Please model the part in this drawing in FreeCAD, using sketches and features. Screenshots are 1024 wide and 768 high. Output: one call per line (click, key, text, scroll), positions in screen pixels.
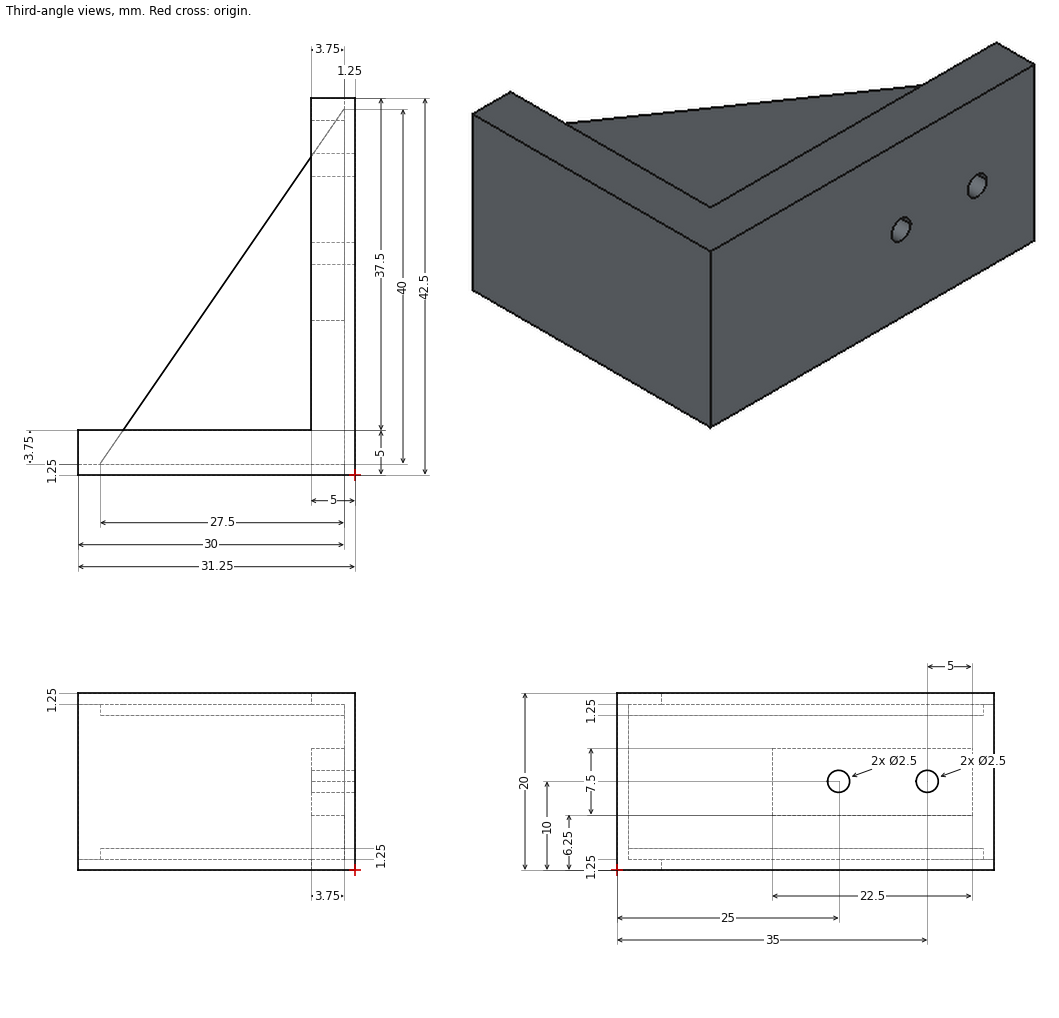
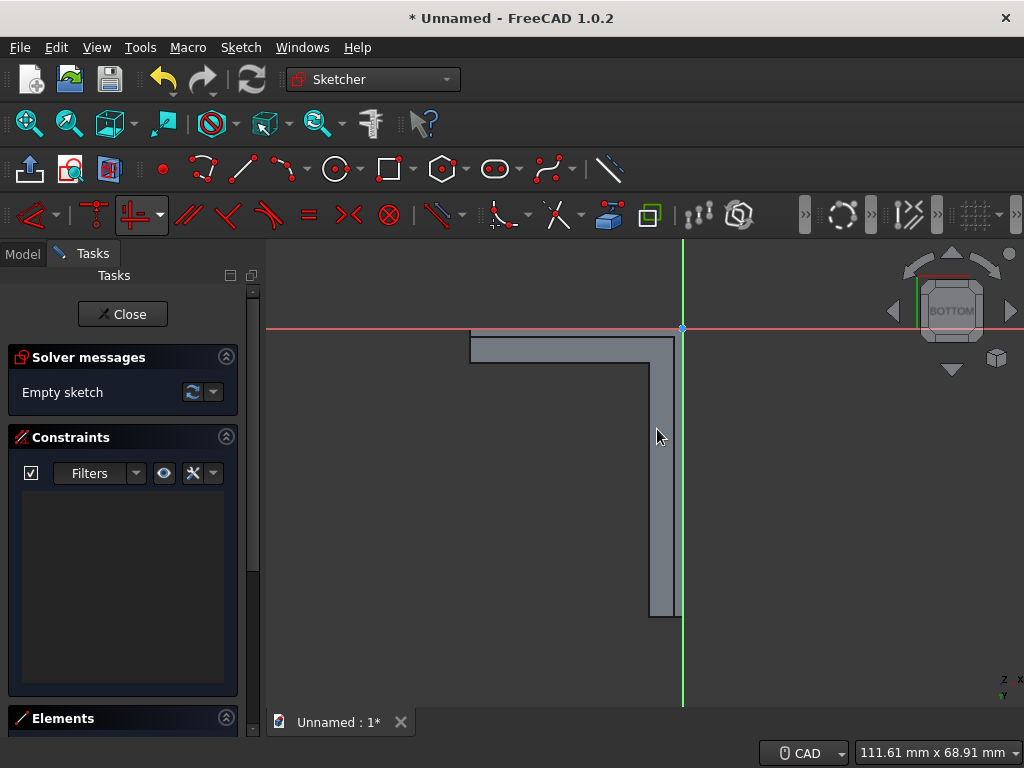
click(204, 170)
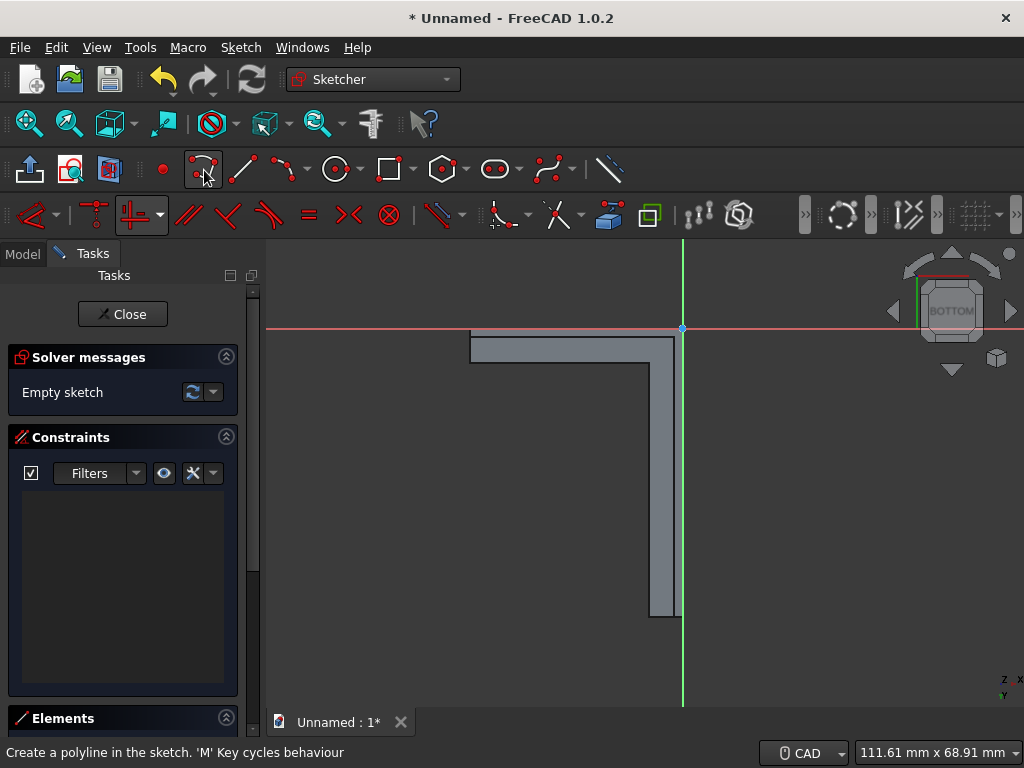
click(683, 329)
click(470, 338)
click(470, 363)
click(649, 363)
click(649, 617)
click(674, 617)
click(683, 329)
key(Escape)
key(Escape)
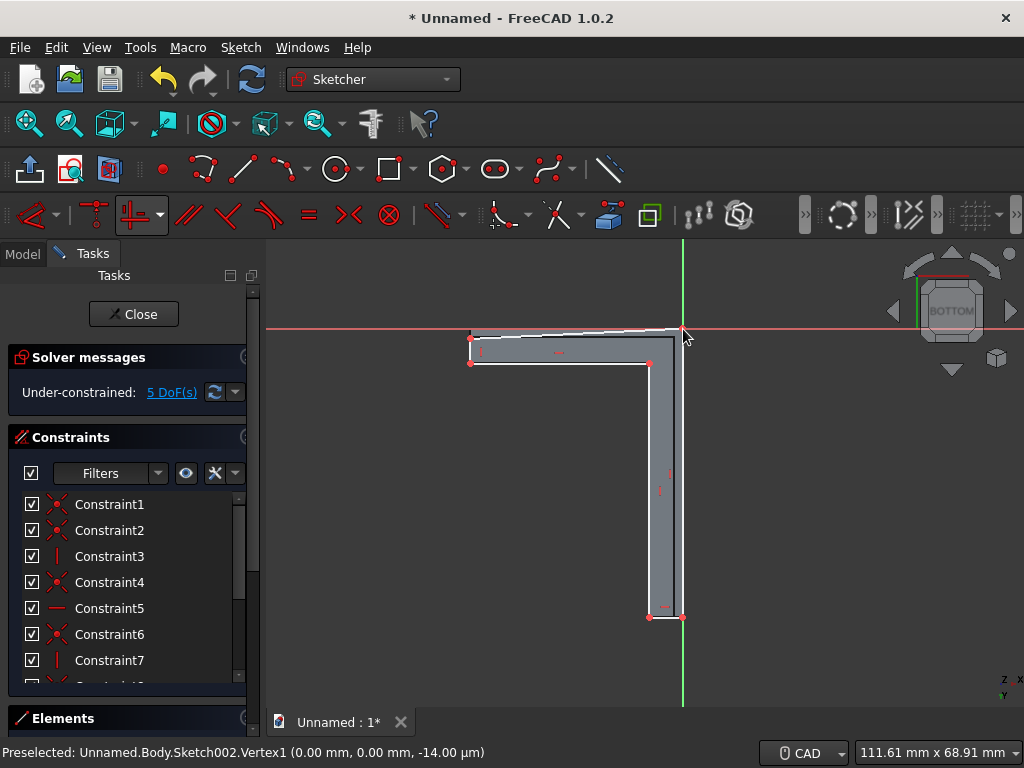
click(619, 332)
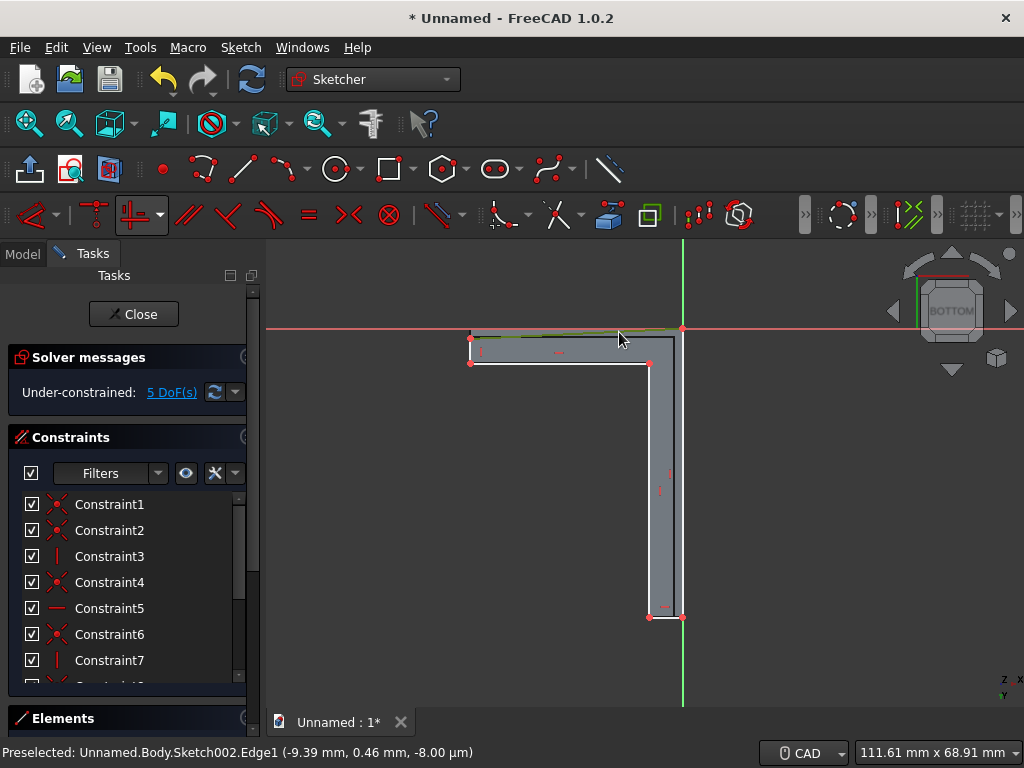
click(162, 216)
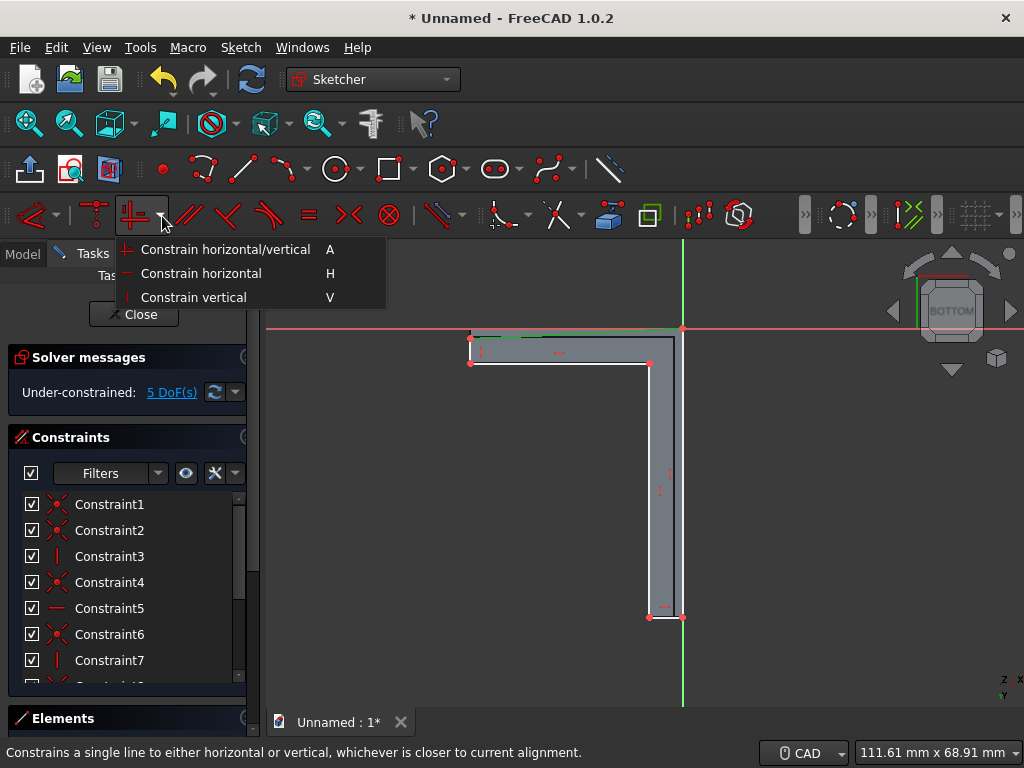
click(251, 273)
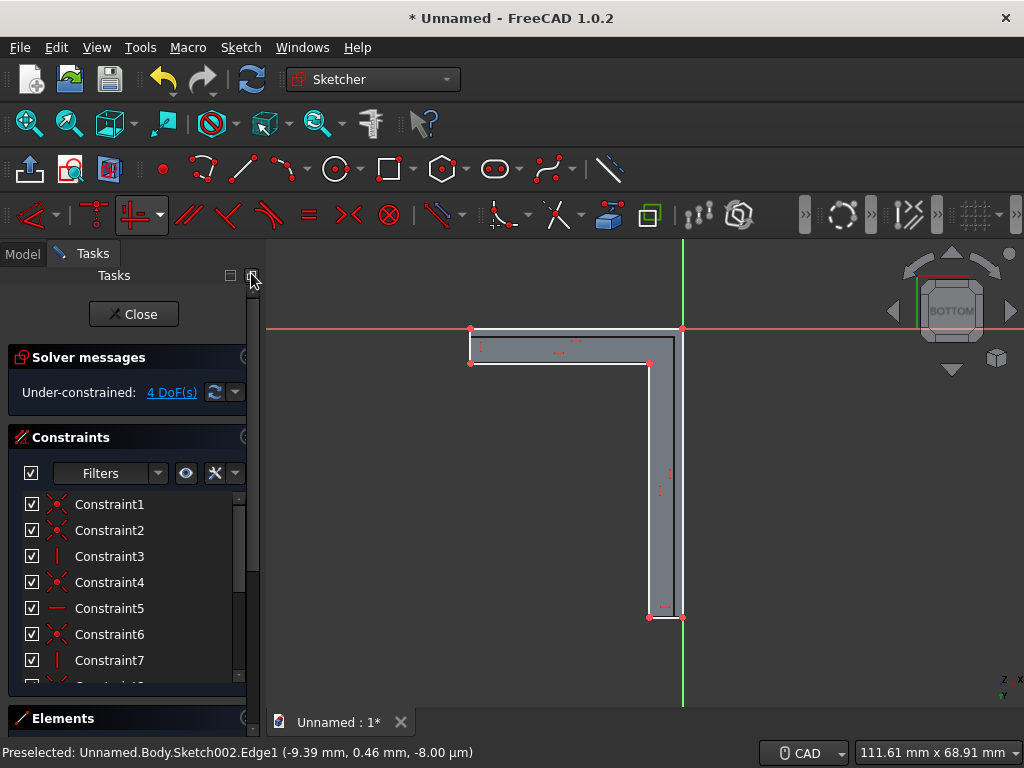
click(32, 216)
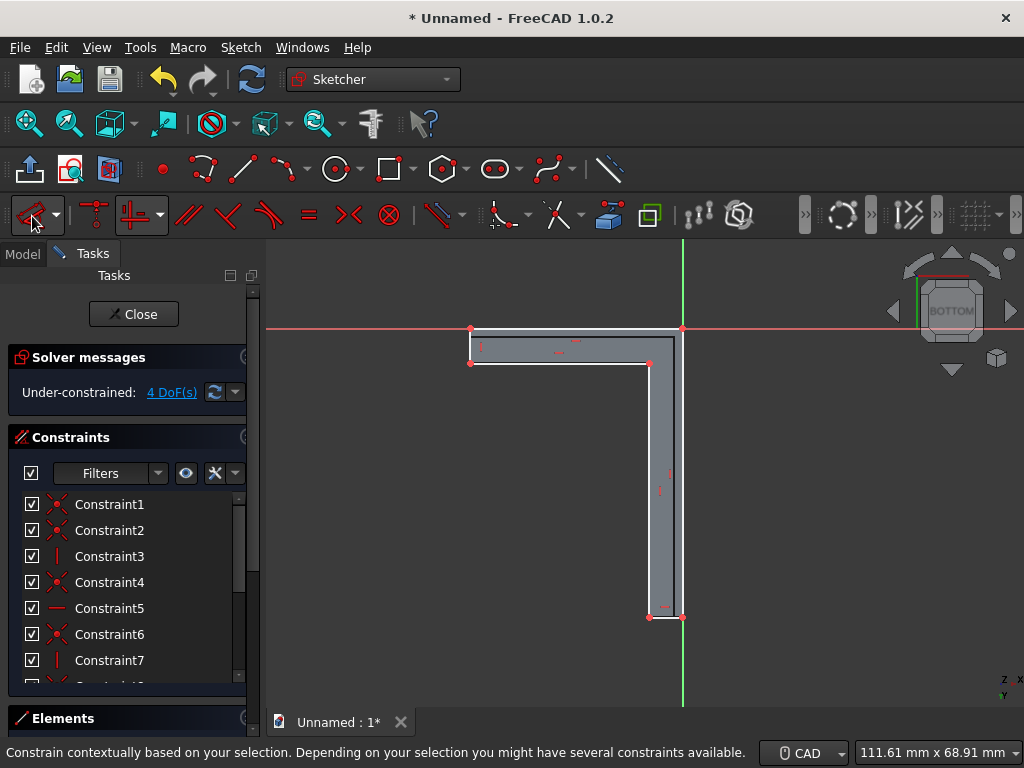
scroll(470, 339, up, 2)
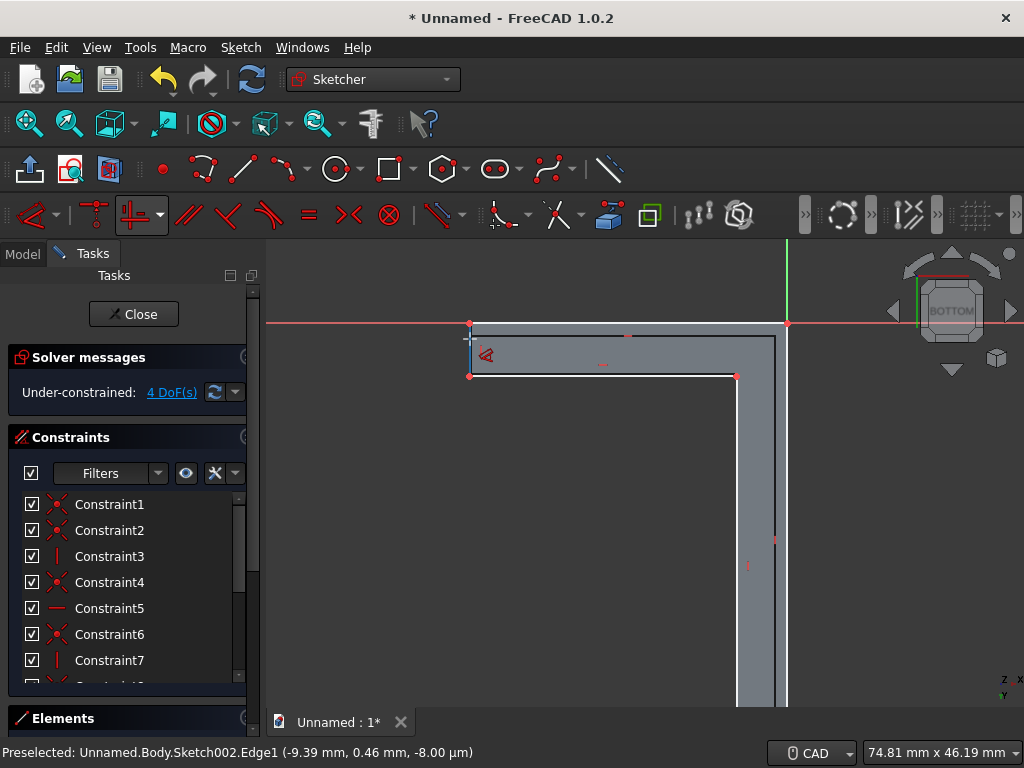
click(470, 339)
click(436, 350)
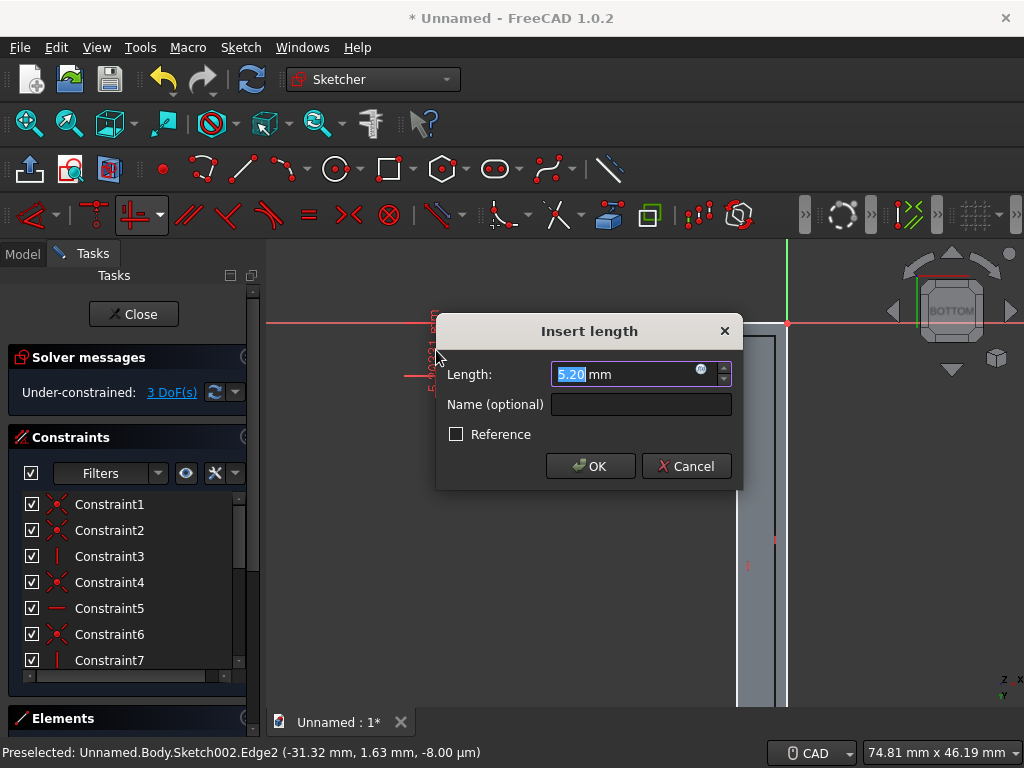
text(5)
key(Return)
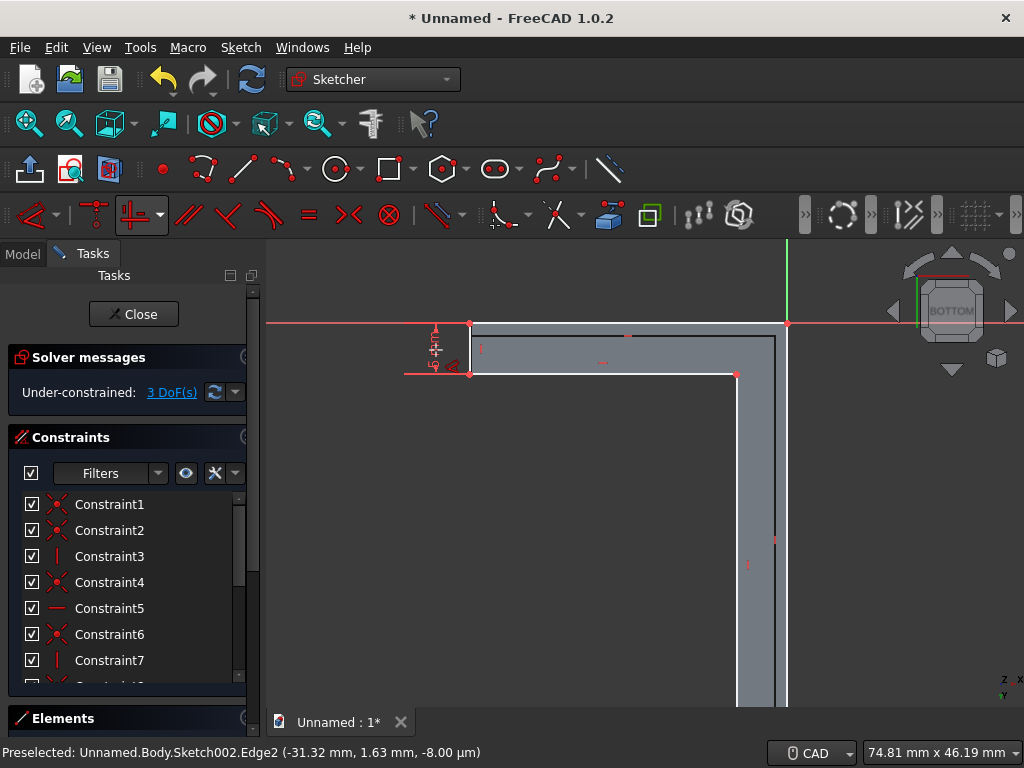
scroll(470, 339, down, 2)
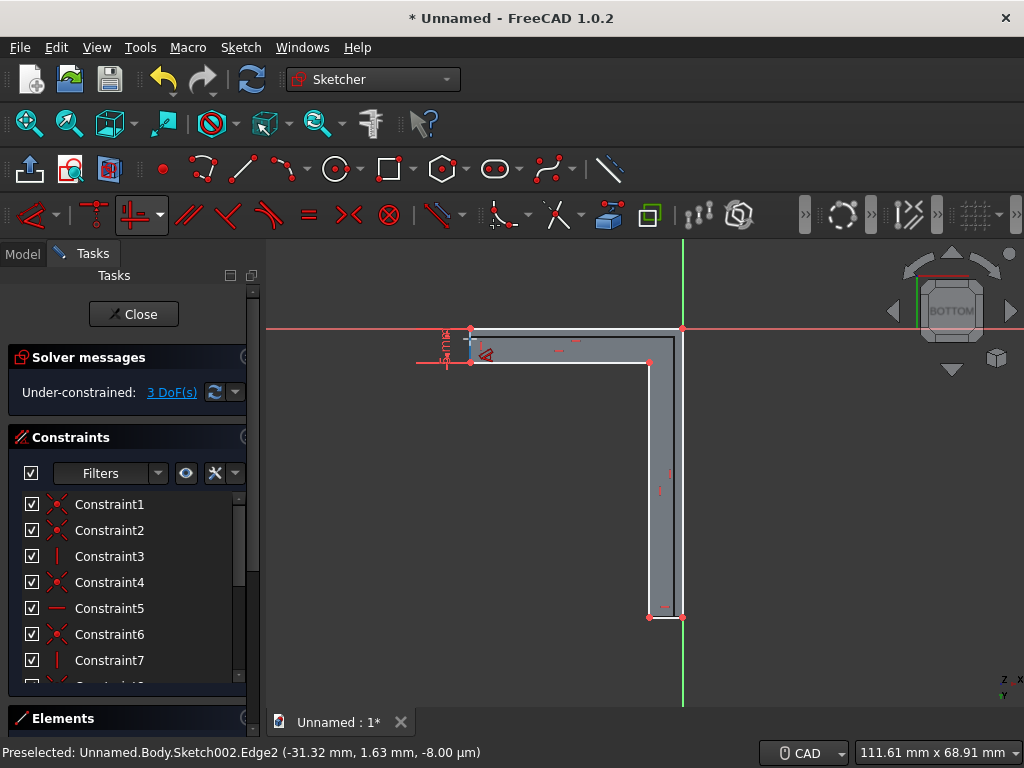
scroll(659, 618, up, 2)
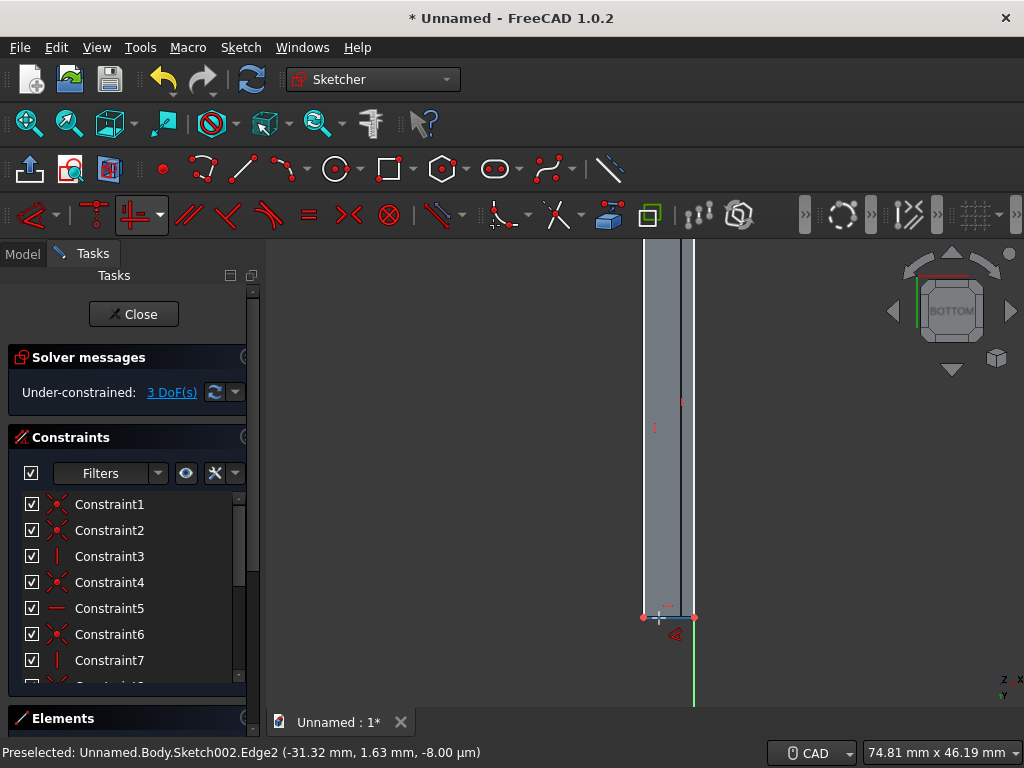
click(659, 618)
click(669, 652)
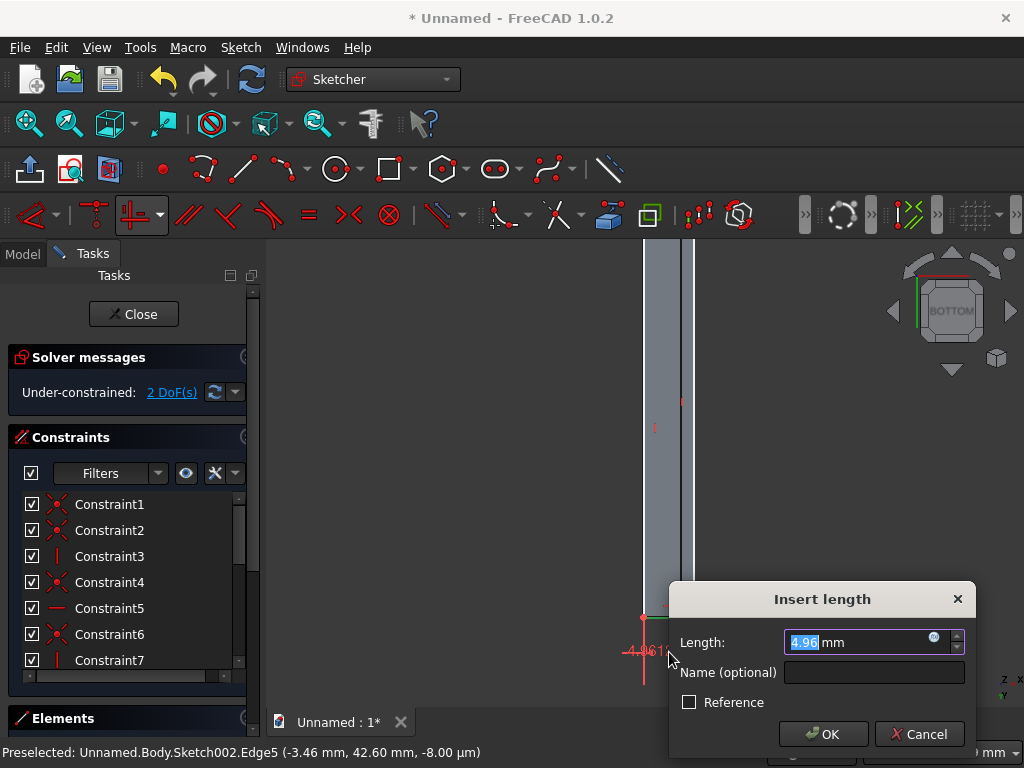
text(5)
key(Return)